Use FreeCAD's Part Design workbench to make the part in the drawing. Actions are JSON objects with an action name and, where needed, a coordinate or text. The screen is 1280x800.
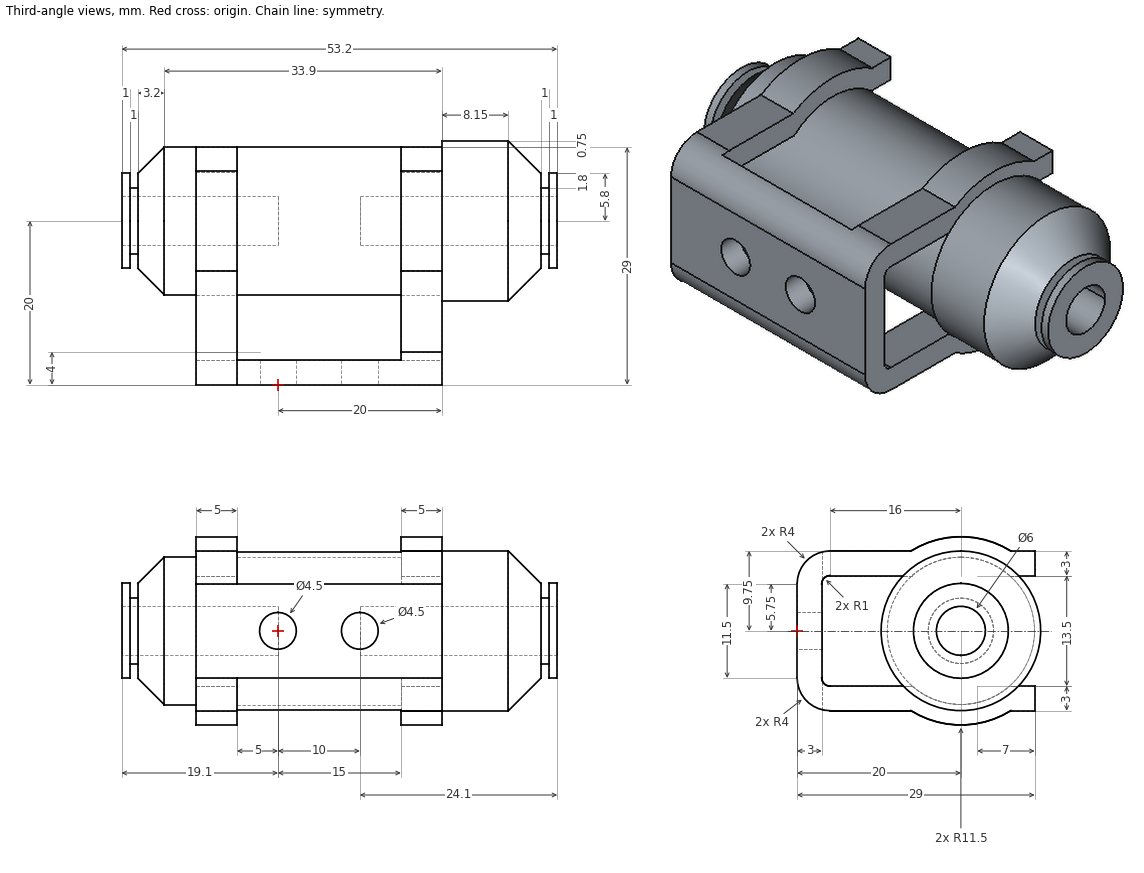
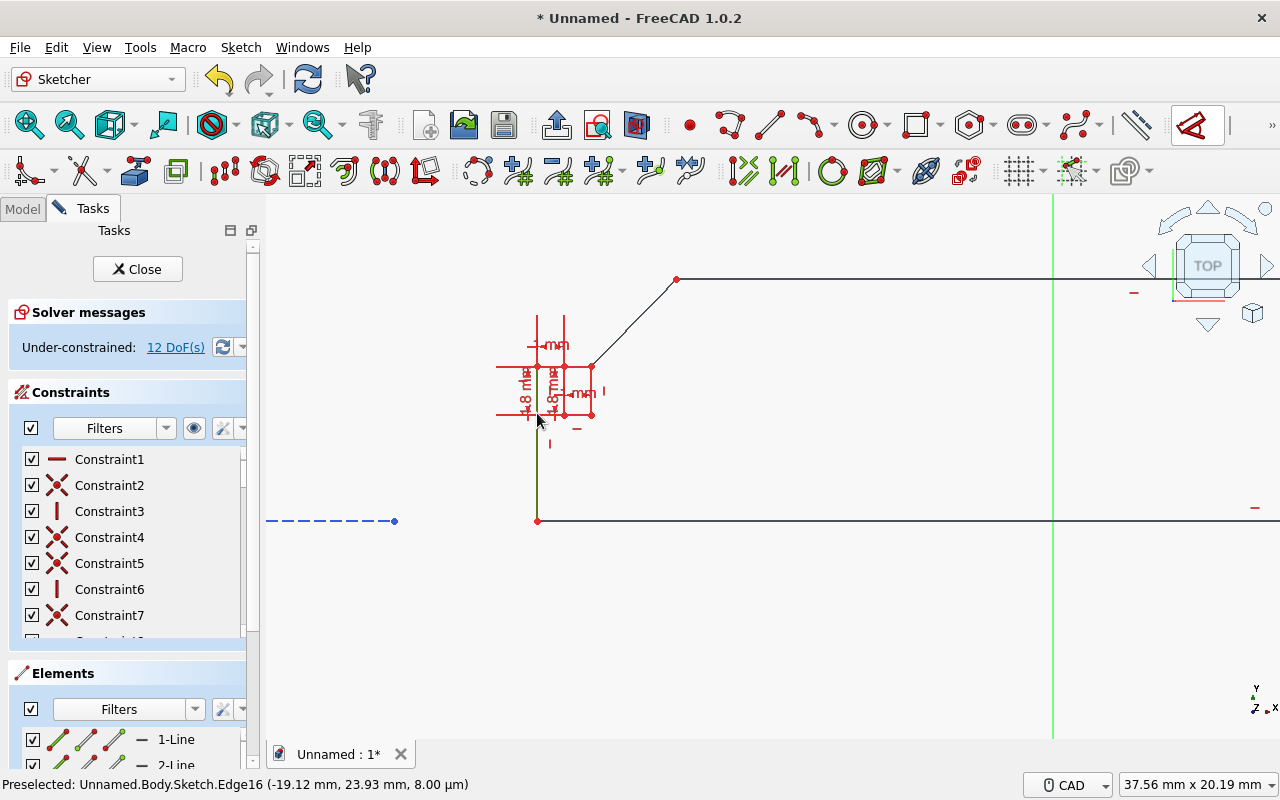
{"action": "left_click", "coordinate": [1218, 126]}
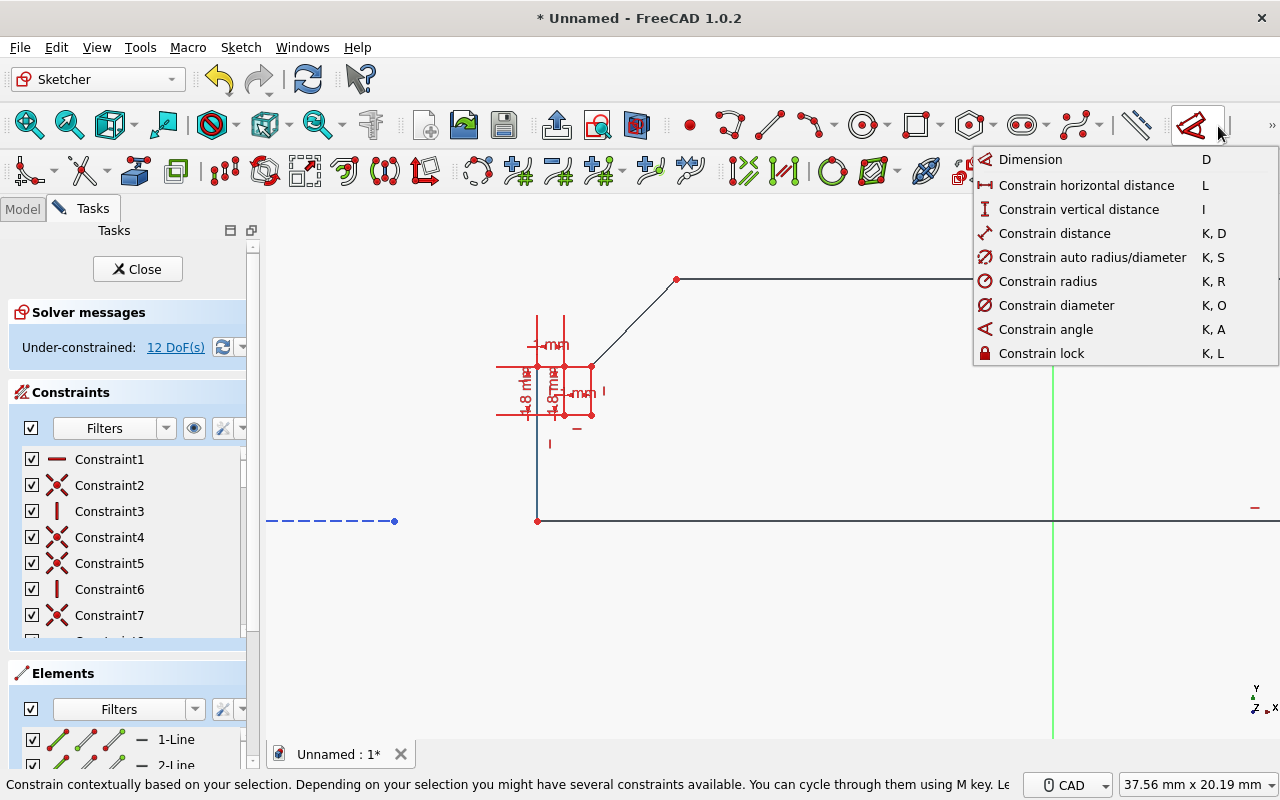
{"action": "left_click", "coordinate": [1126, 209]}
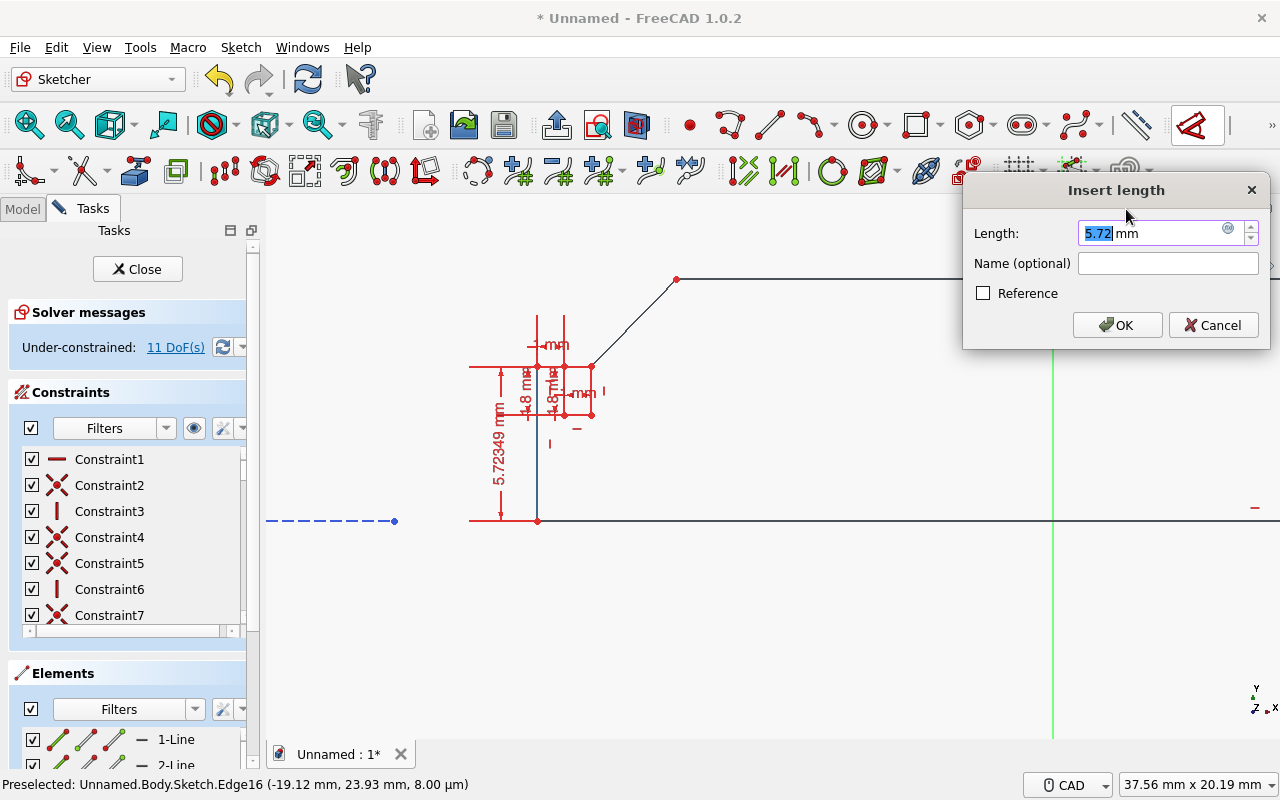
{"action": "type", "text": "5.8"}
{"action": "key", "text": "Return"}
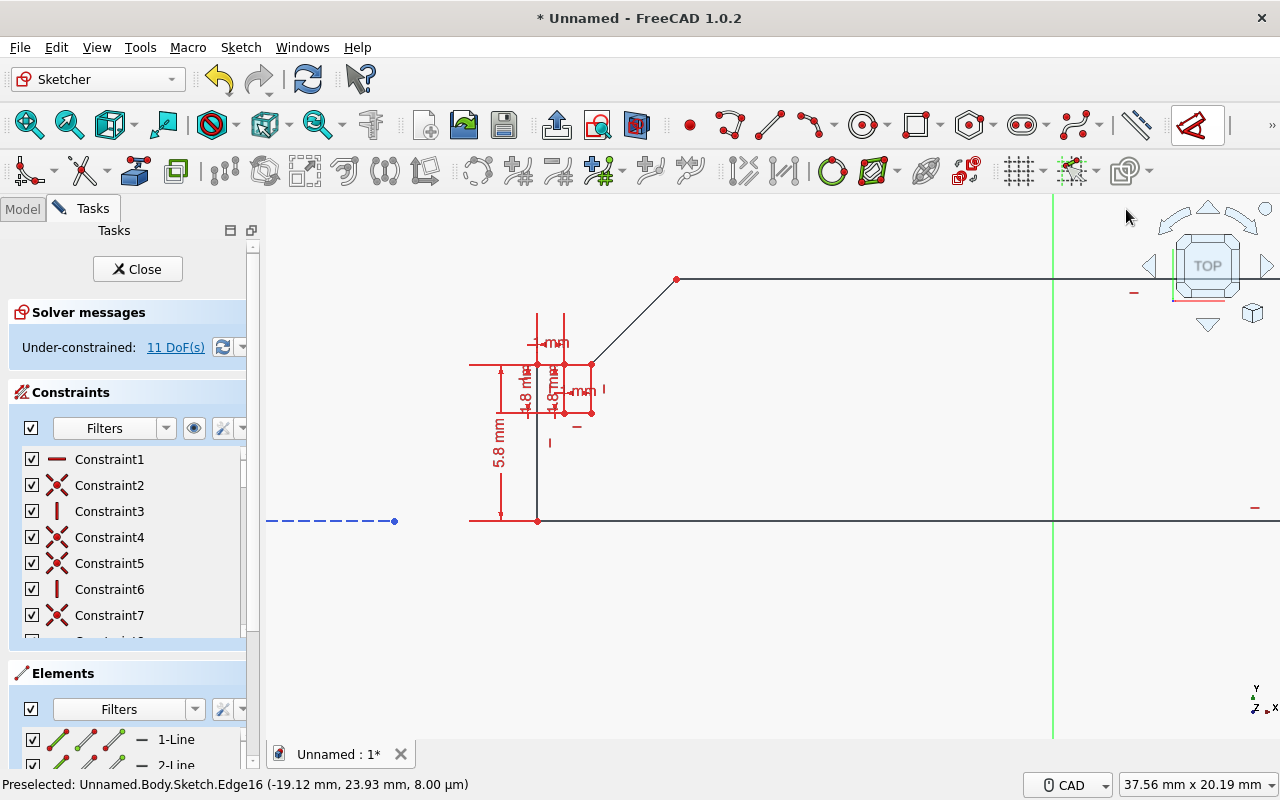
{"action": "left_click", "coordinate": [537, 521]}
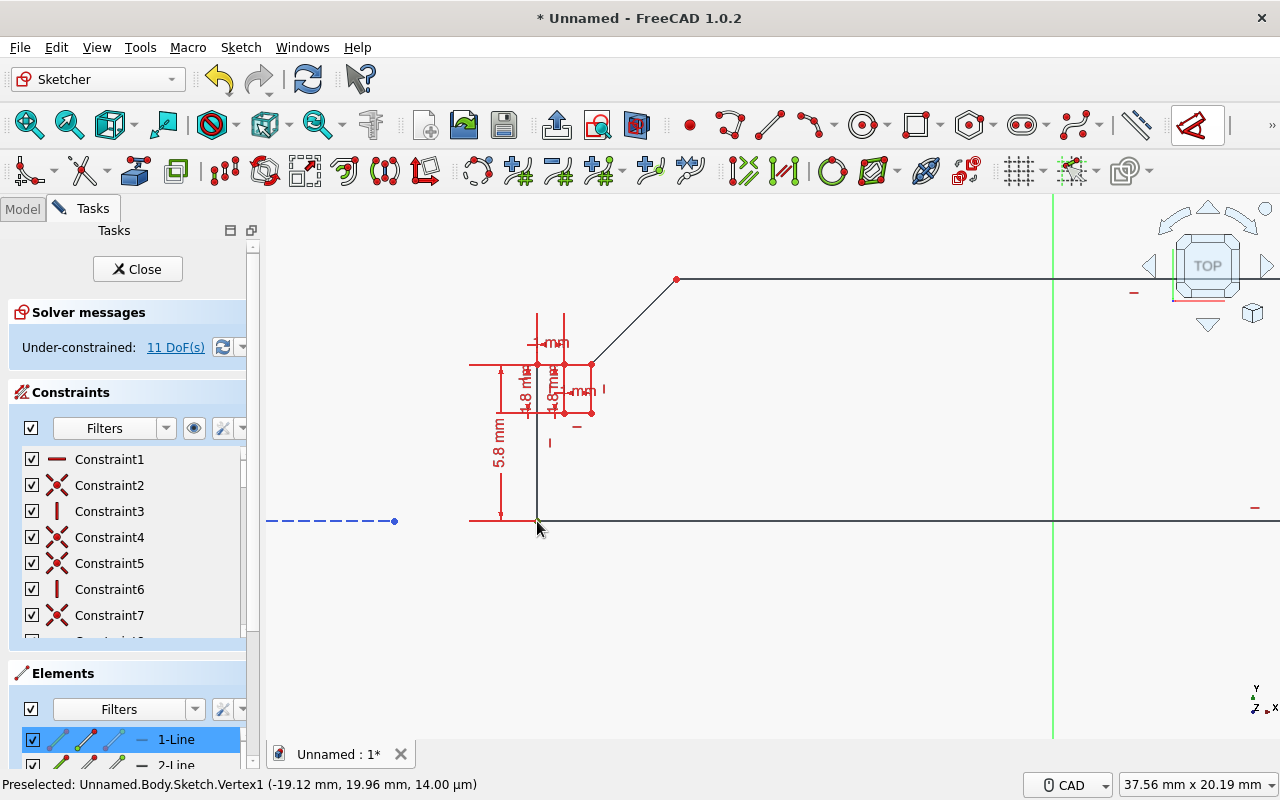
{"action": "left_click", "coordinate": [1218, 126]}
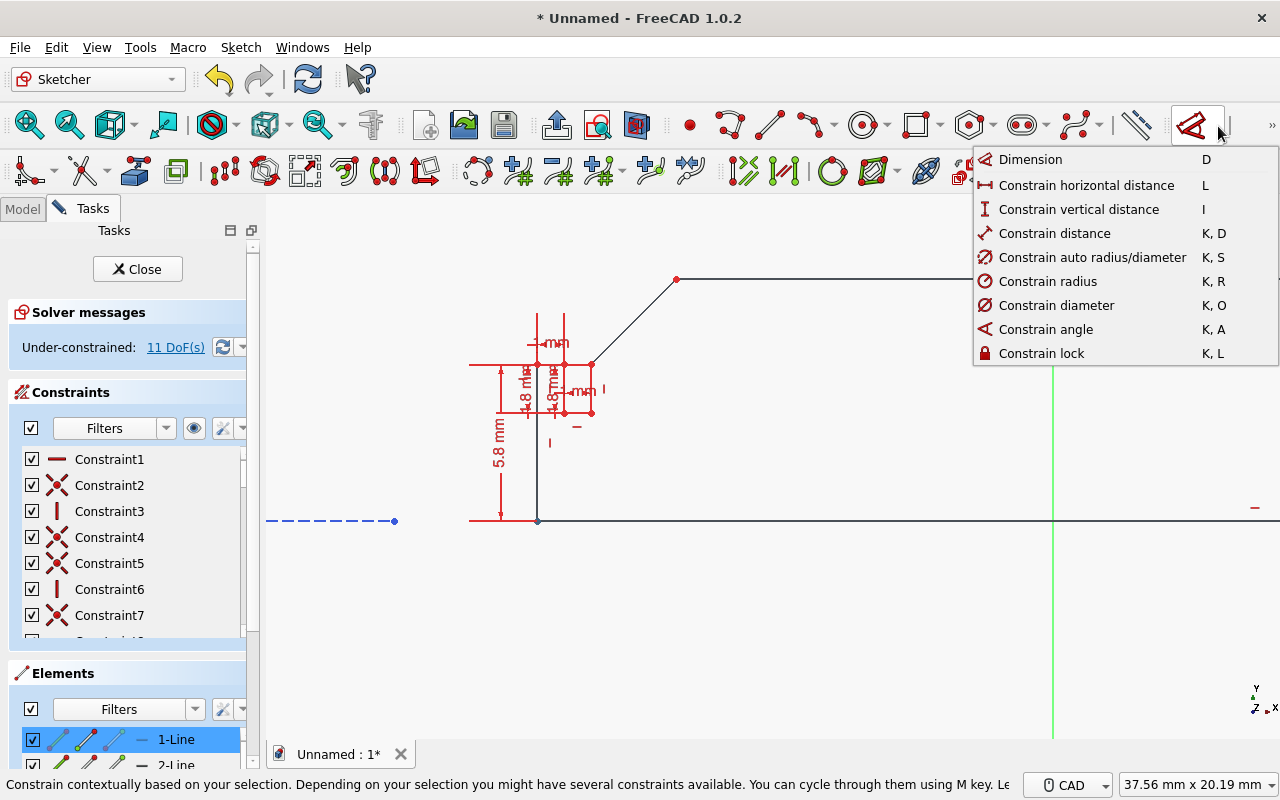
{"action": "left_click", "coordinate": [1126, 209]}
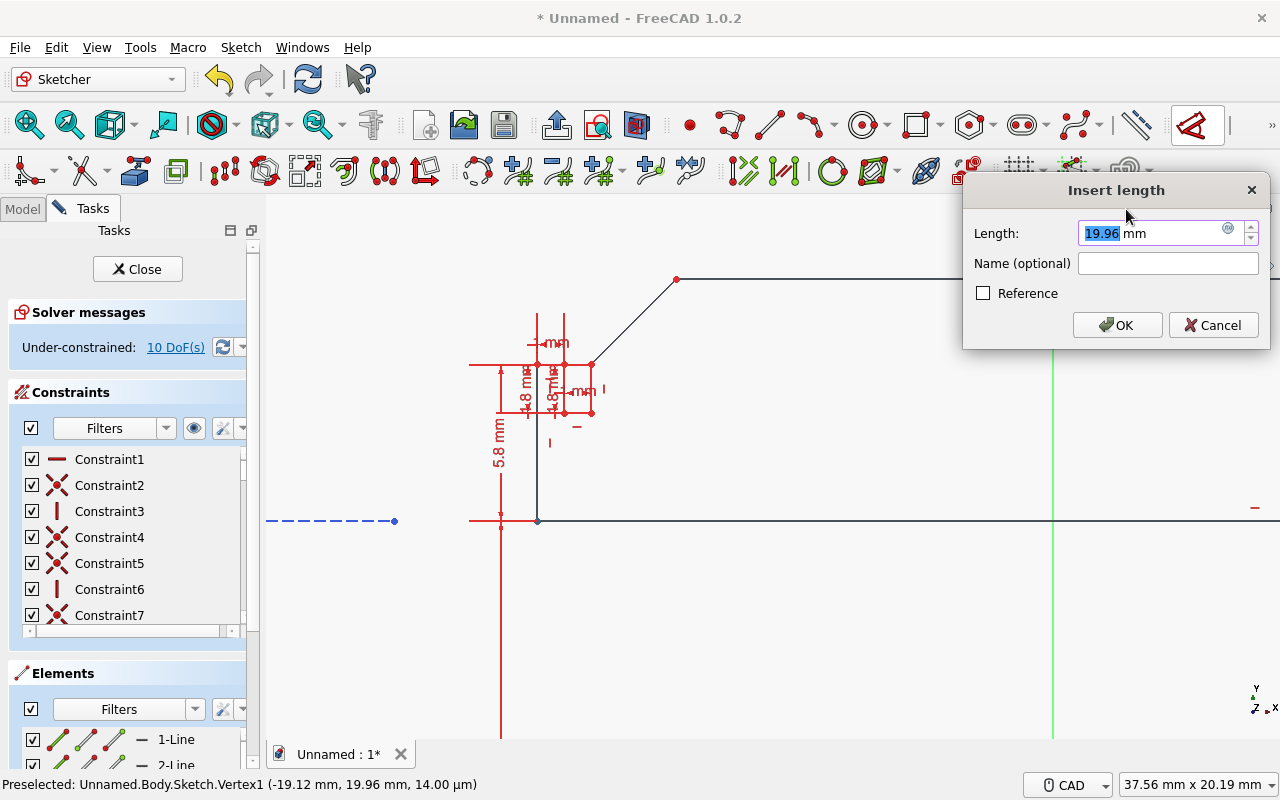
{"action": "type", "text": "20"}
{"action": "key", "text": "Return"}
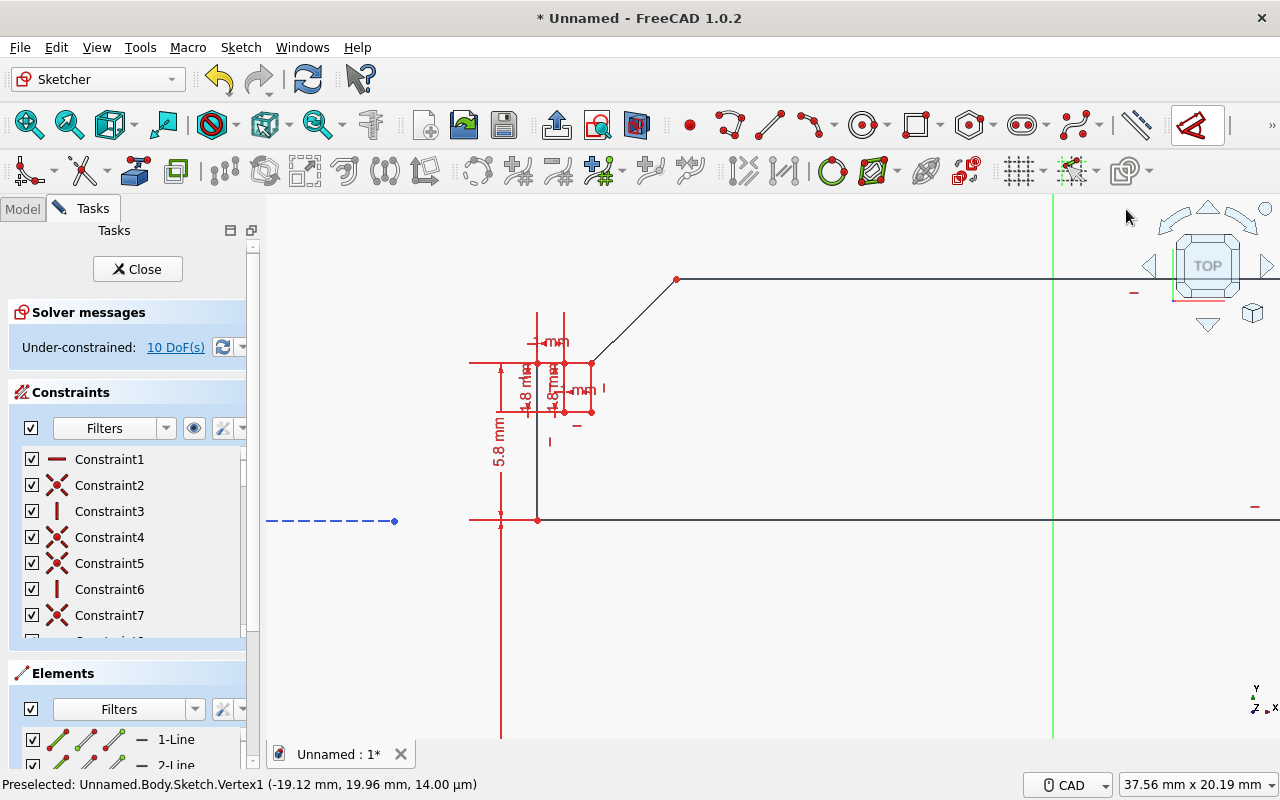
{"action": "scroll", "coordinate": [591, 384], "scroll_direction": "down", "scroll_amount": 6}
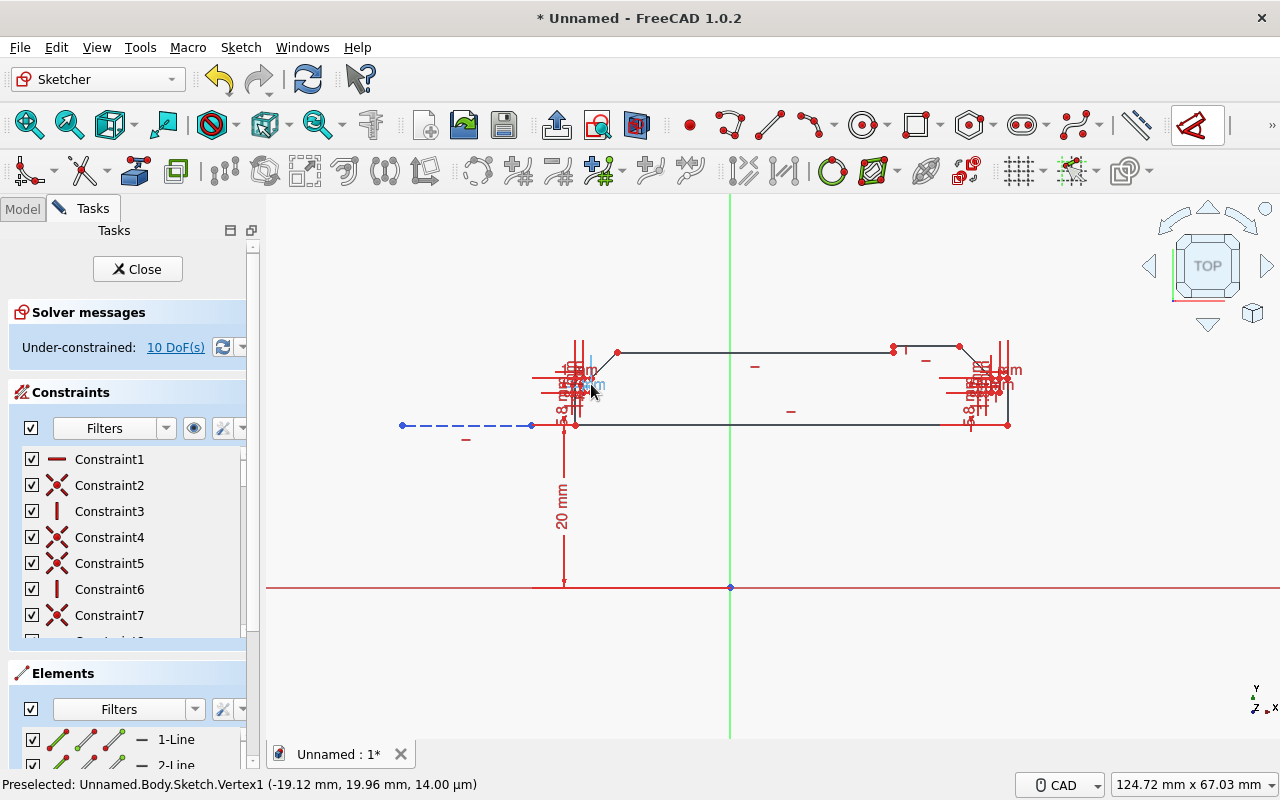
{"action": "scroll", "coordinate": [893, 346], "scroll_direction": "up", "scroll_amount": 4}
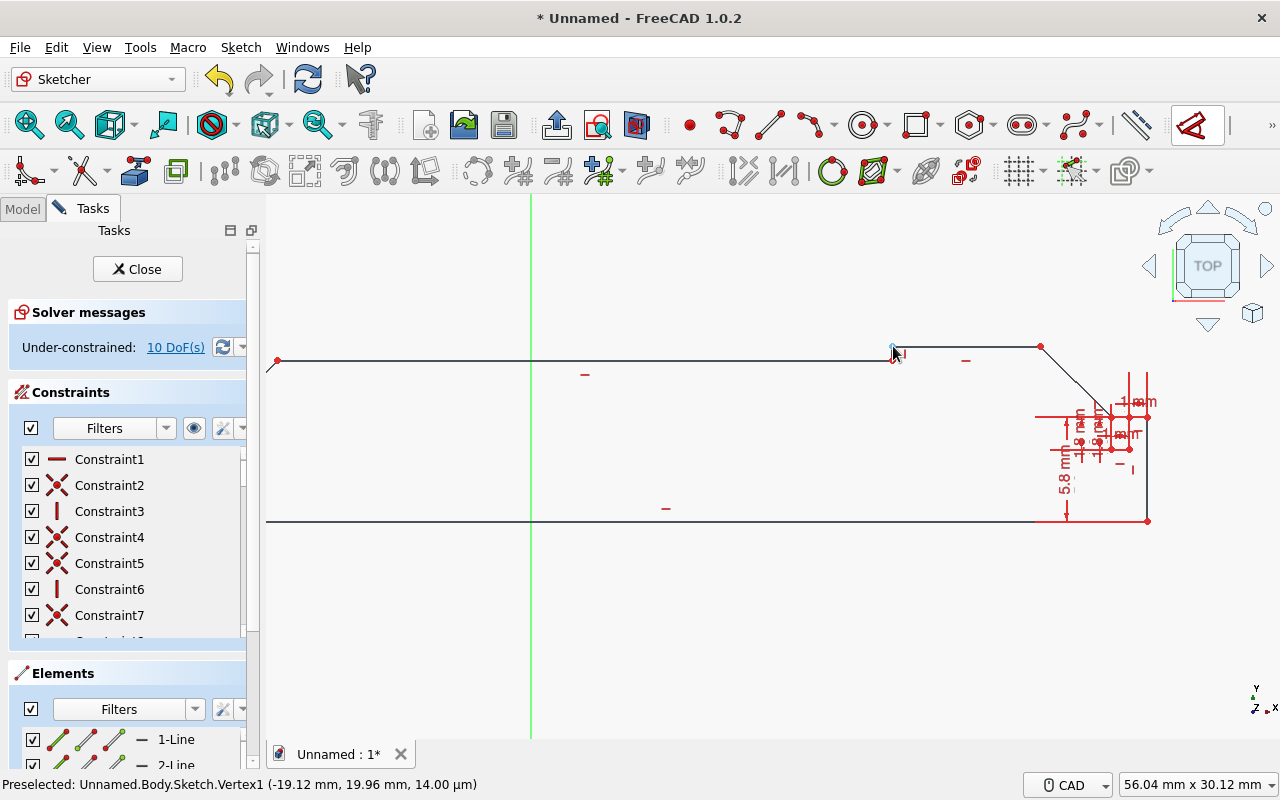
{"action": "left_click", "coordinate": [892, 347]}